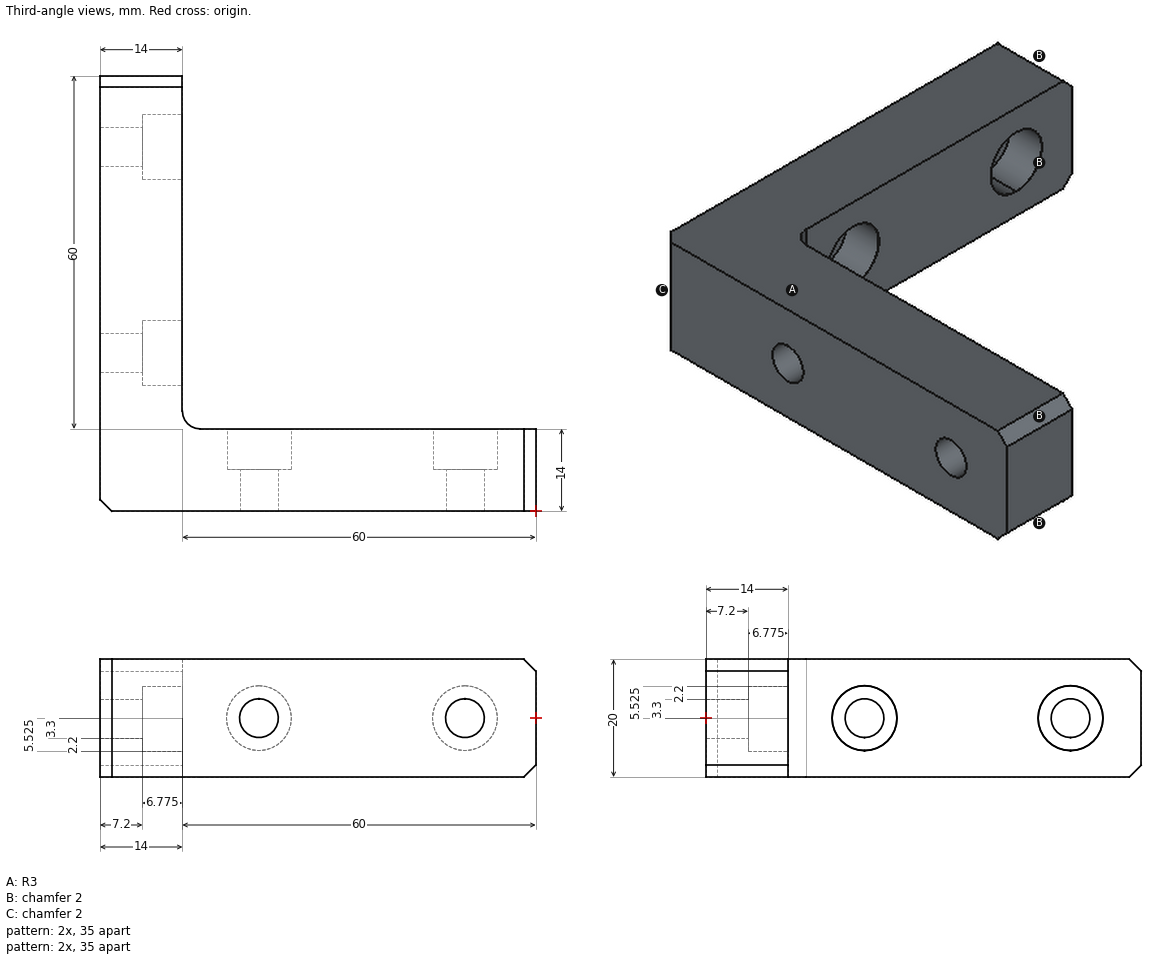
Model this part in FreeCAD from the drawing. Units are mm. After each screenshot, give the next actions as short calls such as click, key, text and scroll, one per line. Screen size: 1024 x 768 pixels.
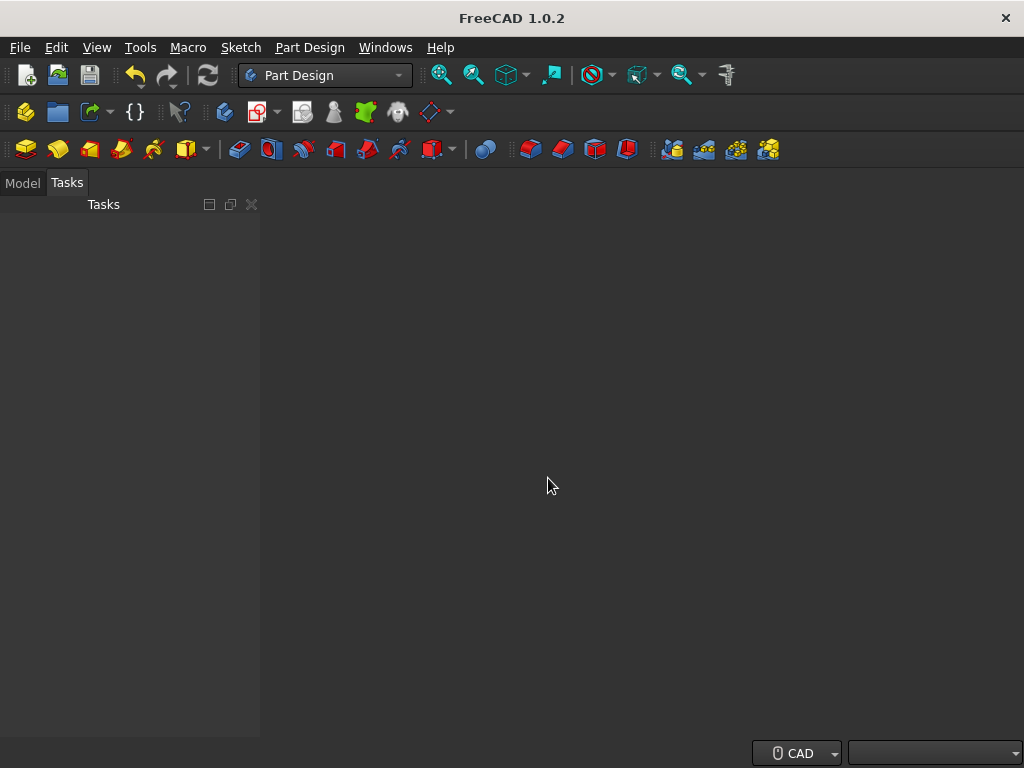
click(26, 76)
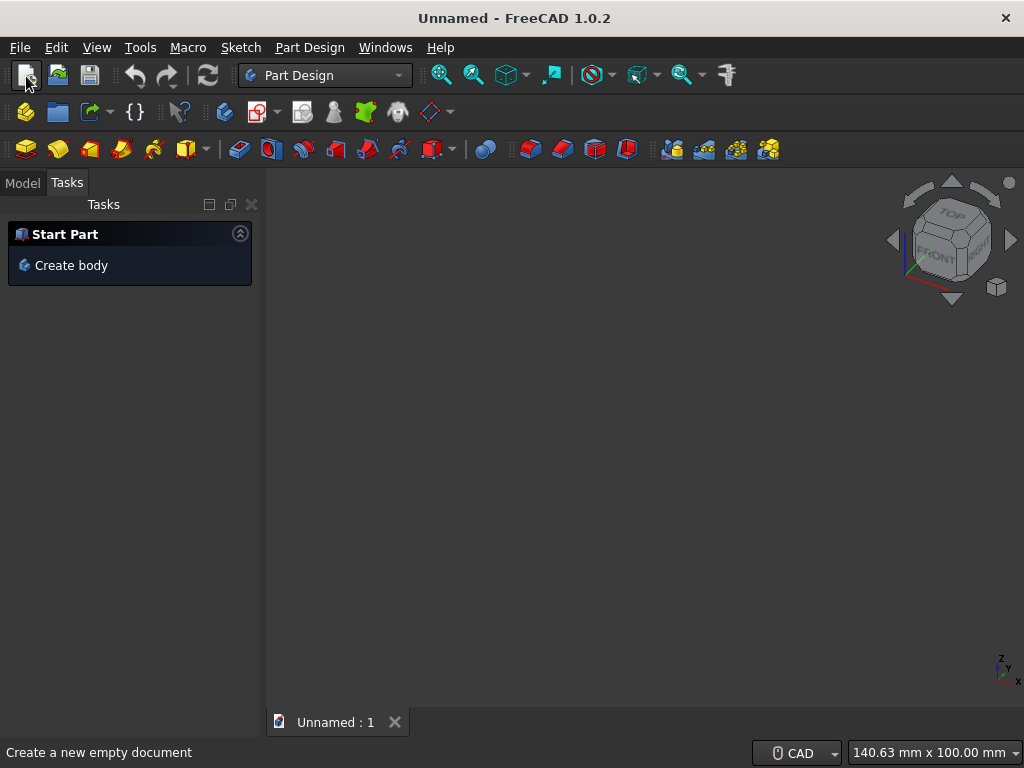
click(258, 112)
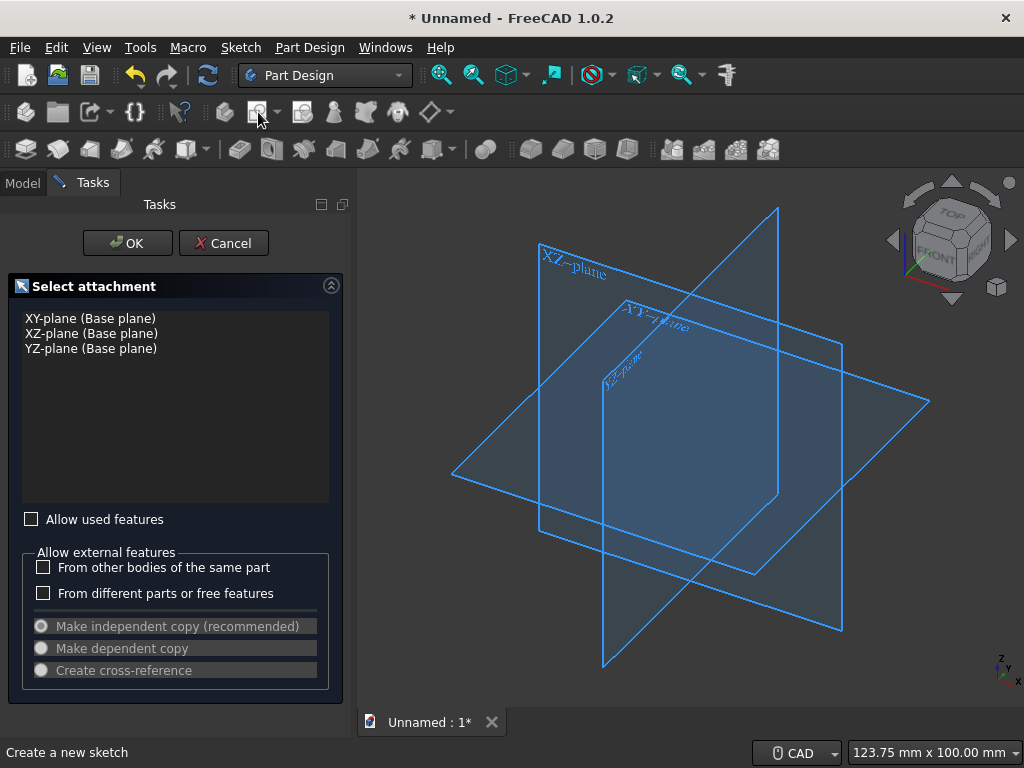
click(82, 318)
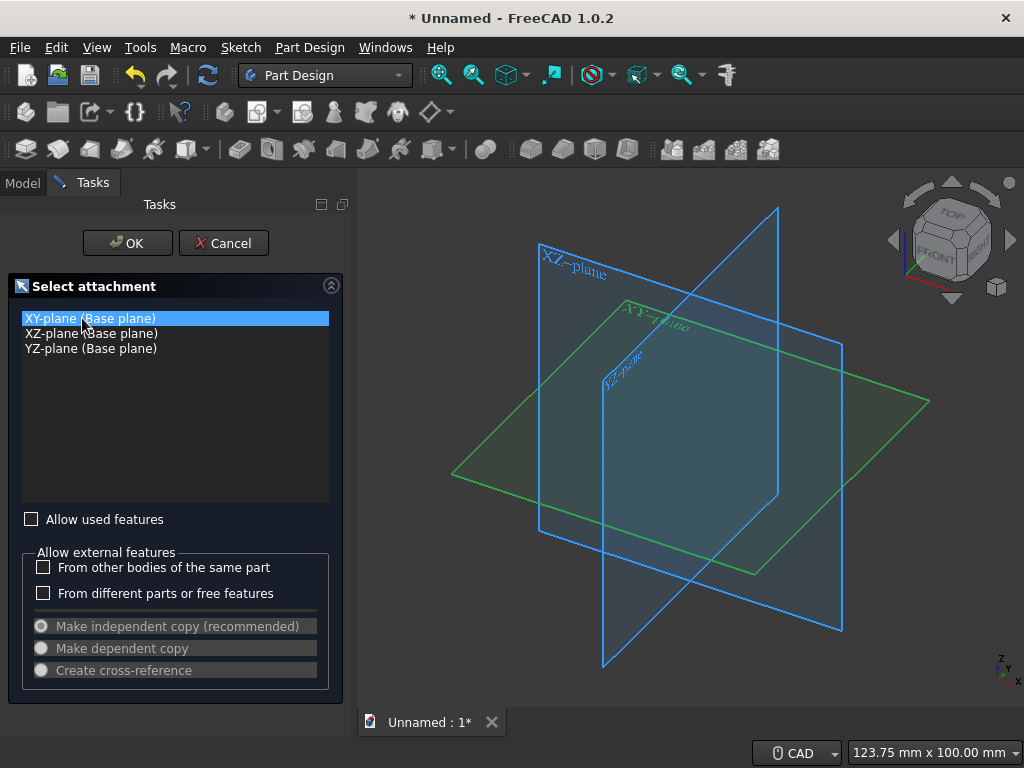
click(128, 243)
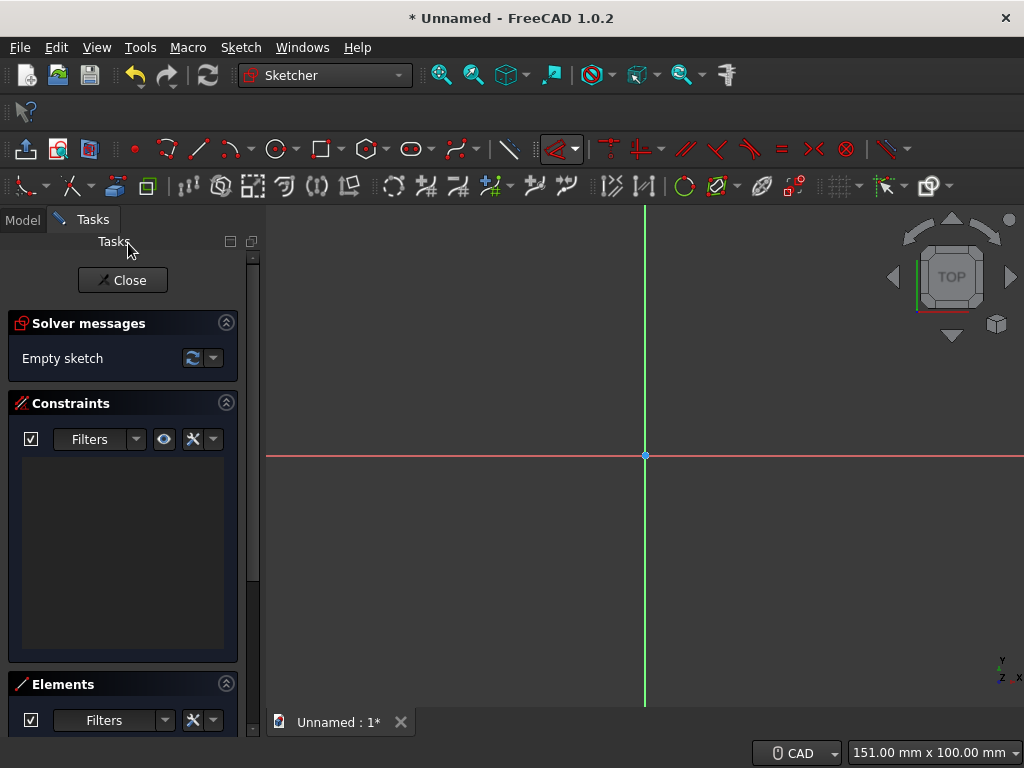
scroll(815, 679, down, 2)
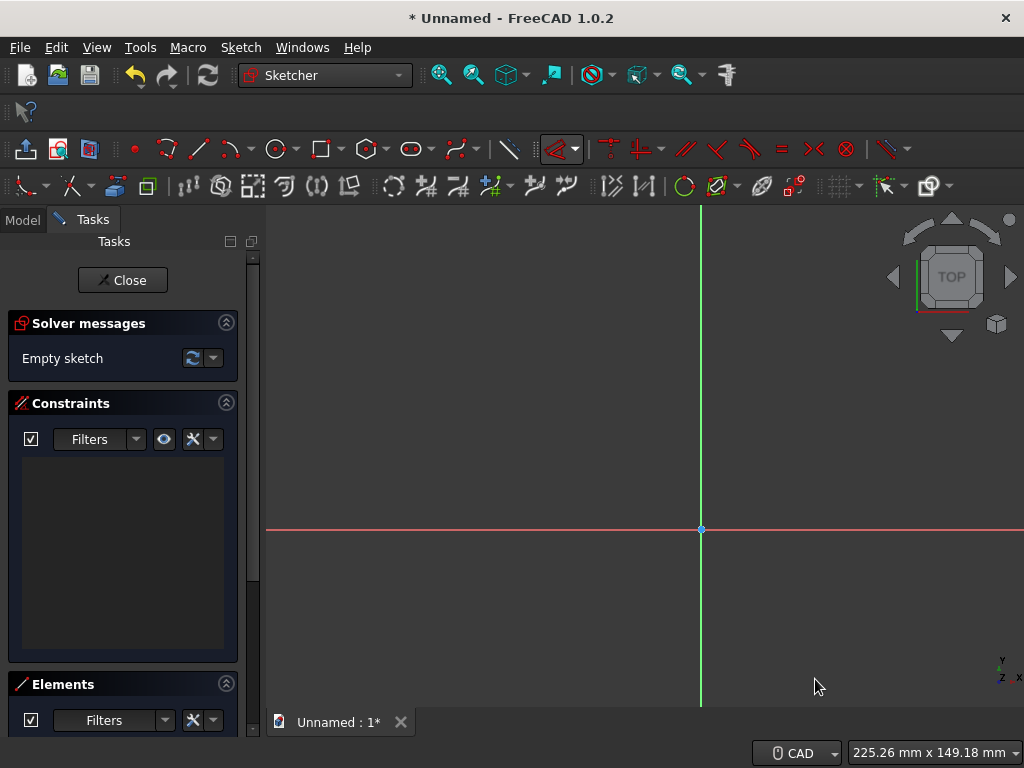
click(168, 150)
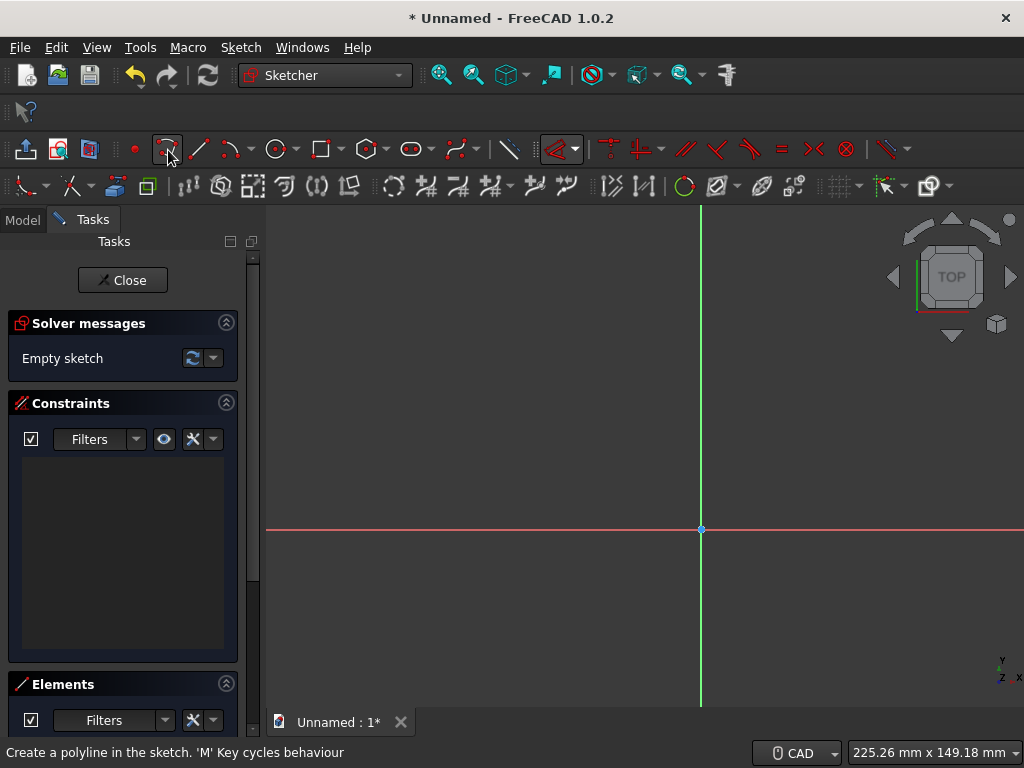
click(701, 530)
click(692, 483)
click(499, 483)
click(499, 281)
click(452, 281)
click(452, 521)
click(701, 530)
key(Escape)
key(Escape)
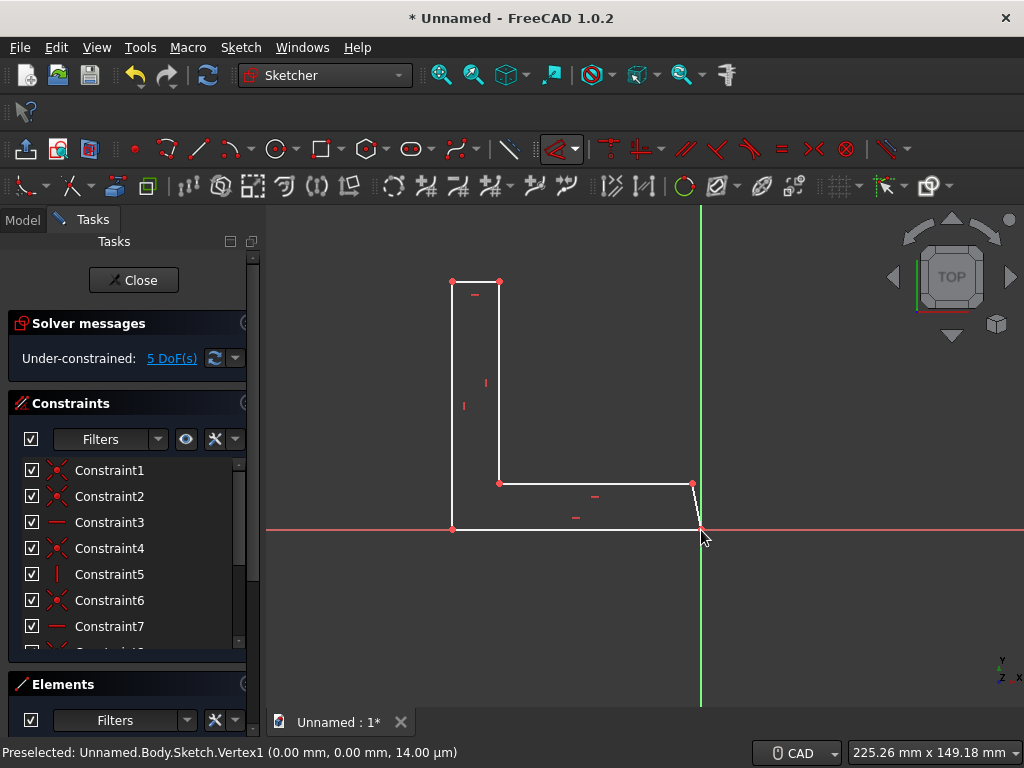
click(698, 516)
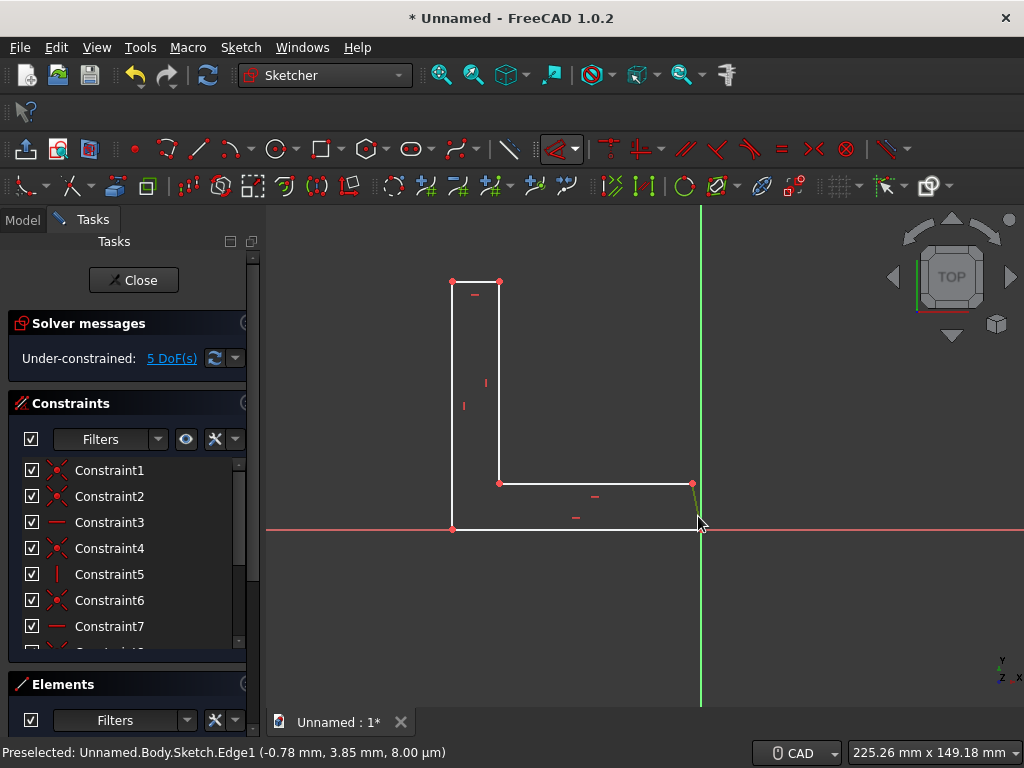
key(v)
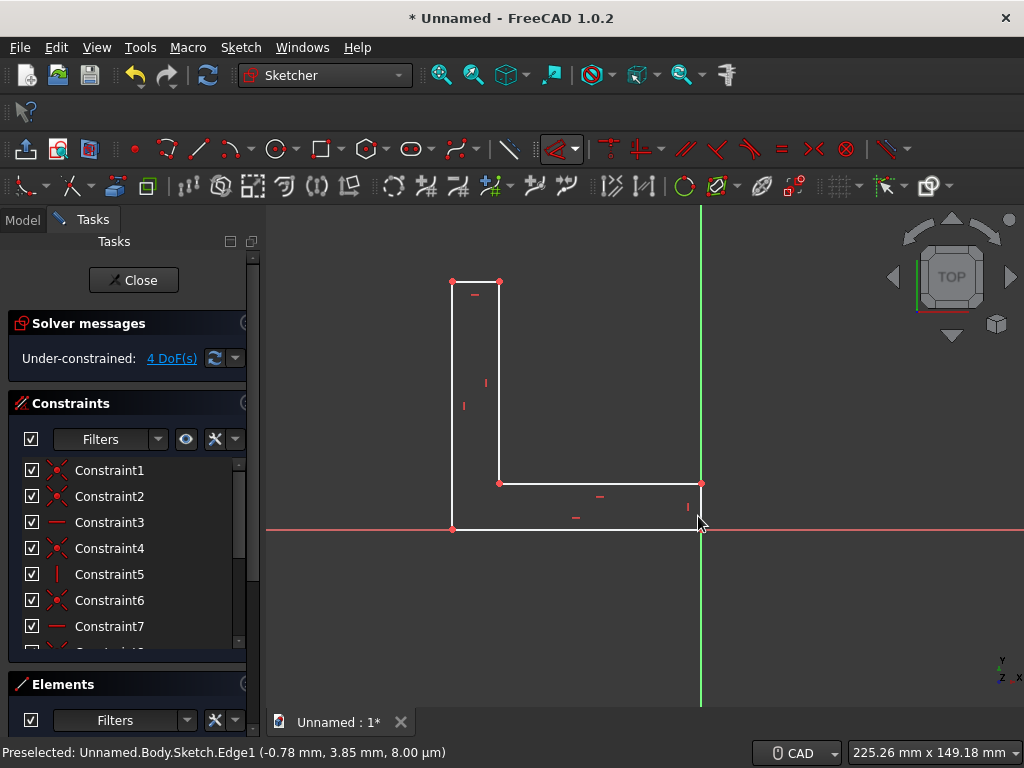
click(701, 516)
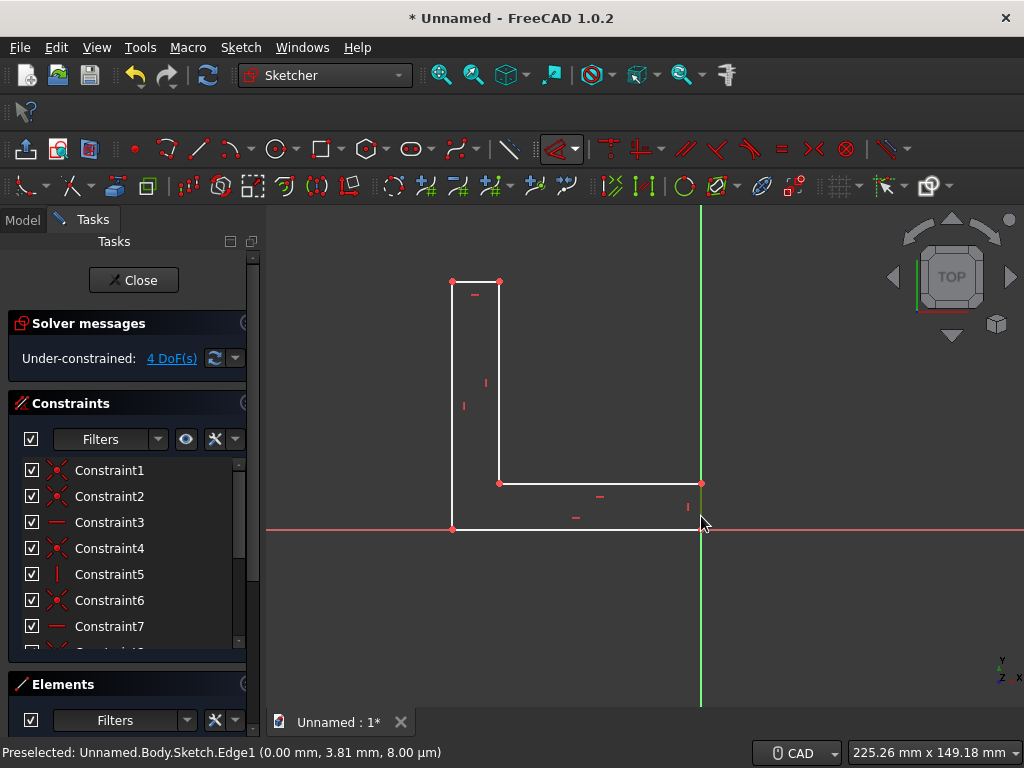
key(i)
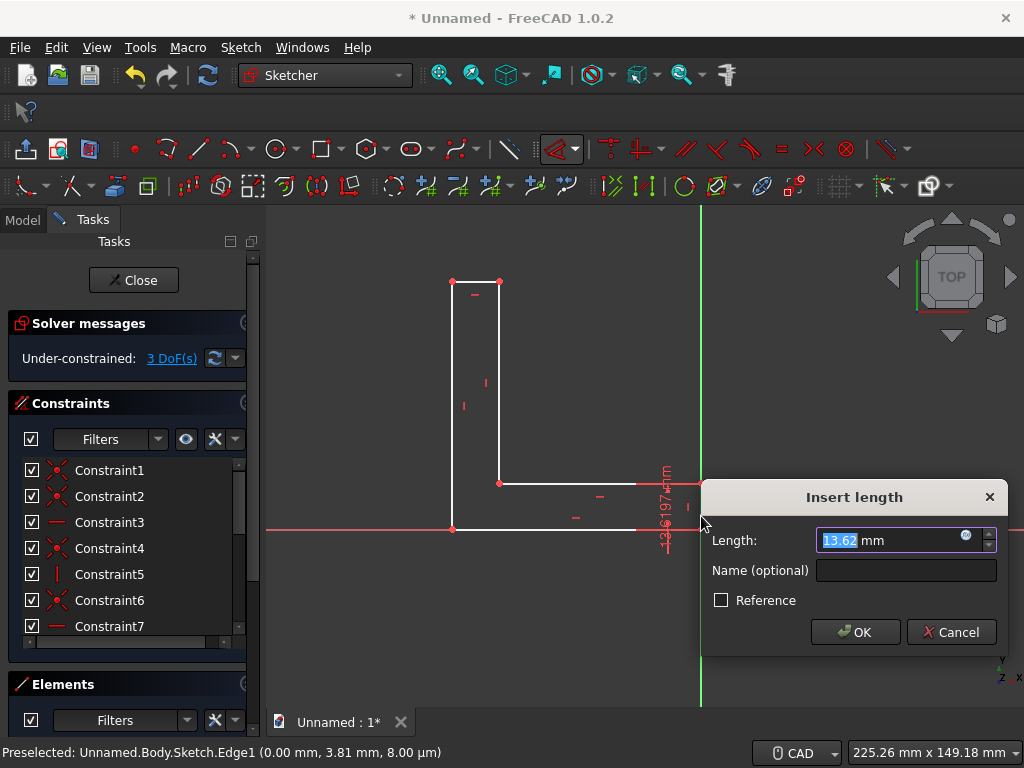
text(14)
key(Return)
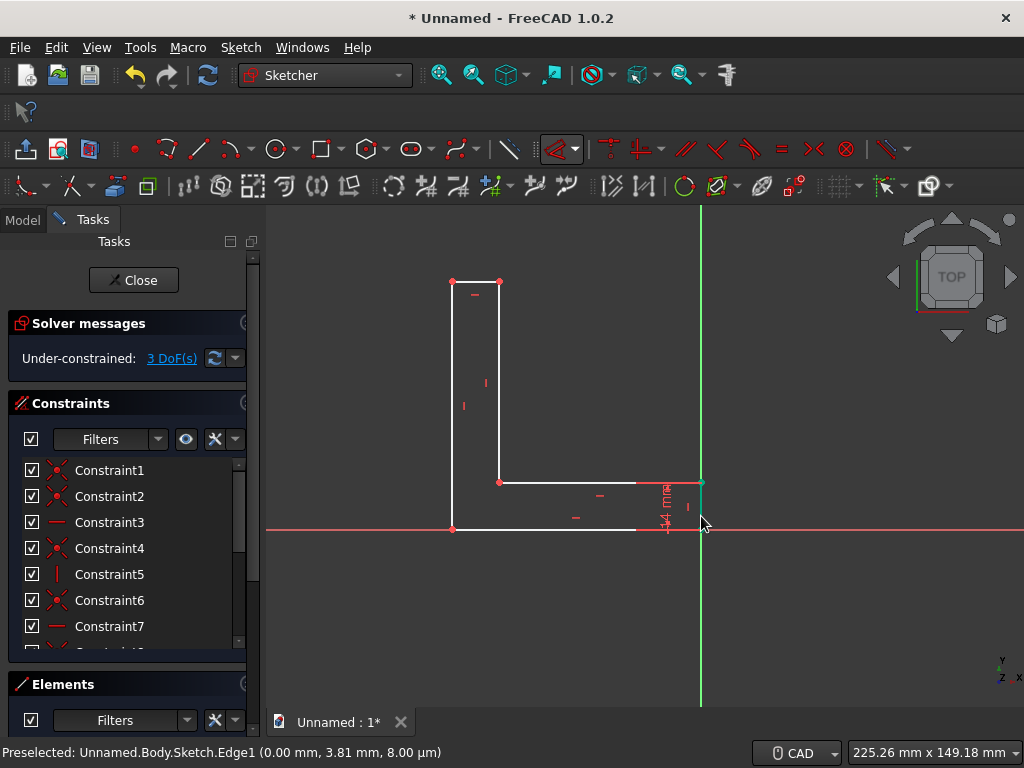
click(641, 483)